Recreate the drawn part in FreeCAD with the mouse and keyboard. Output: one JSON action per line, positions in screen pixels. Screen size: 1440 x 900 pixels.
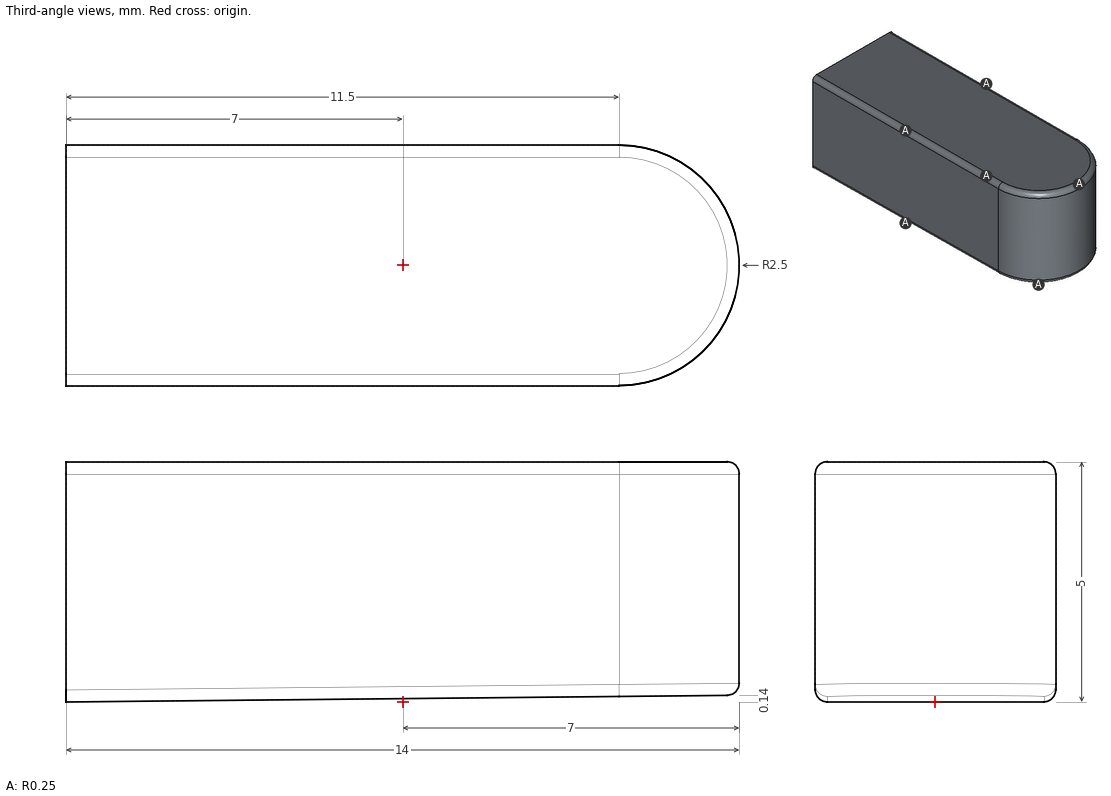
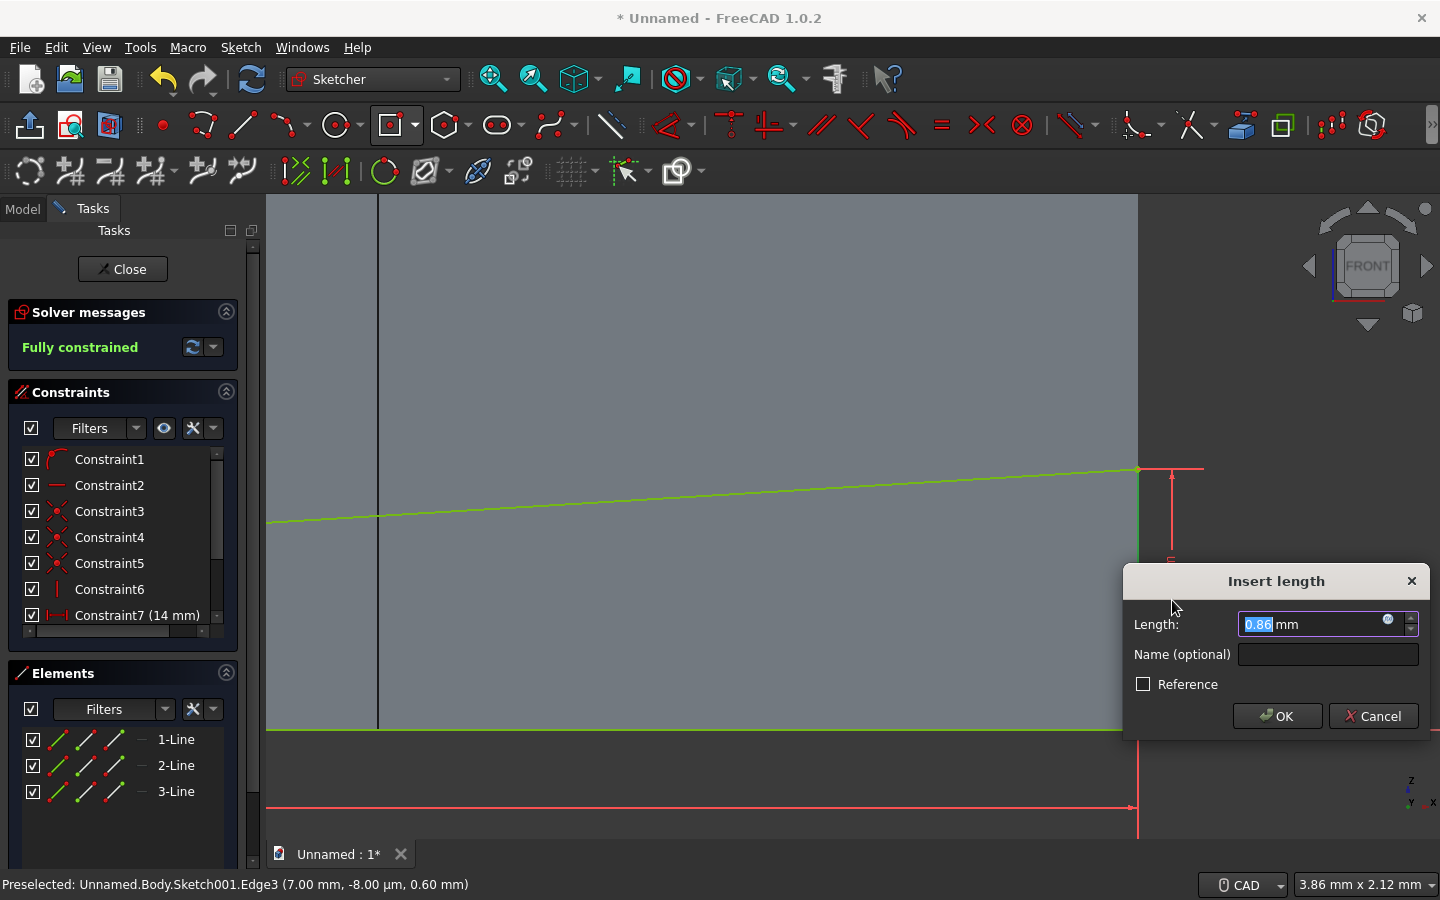
{"action": "type", "text": "0.14"}
{"action": "key", "text": "Return"}
{"action": "key", "text": "Escape"}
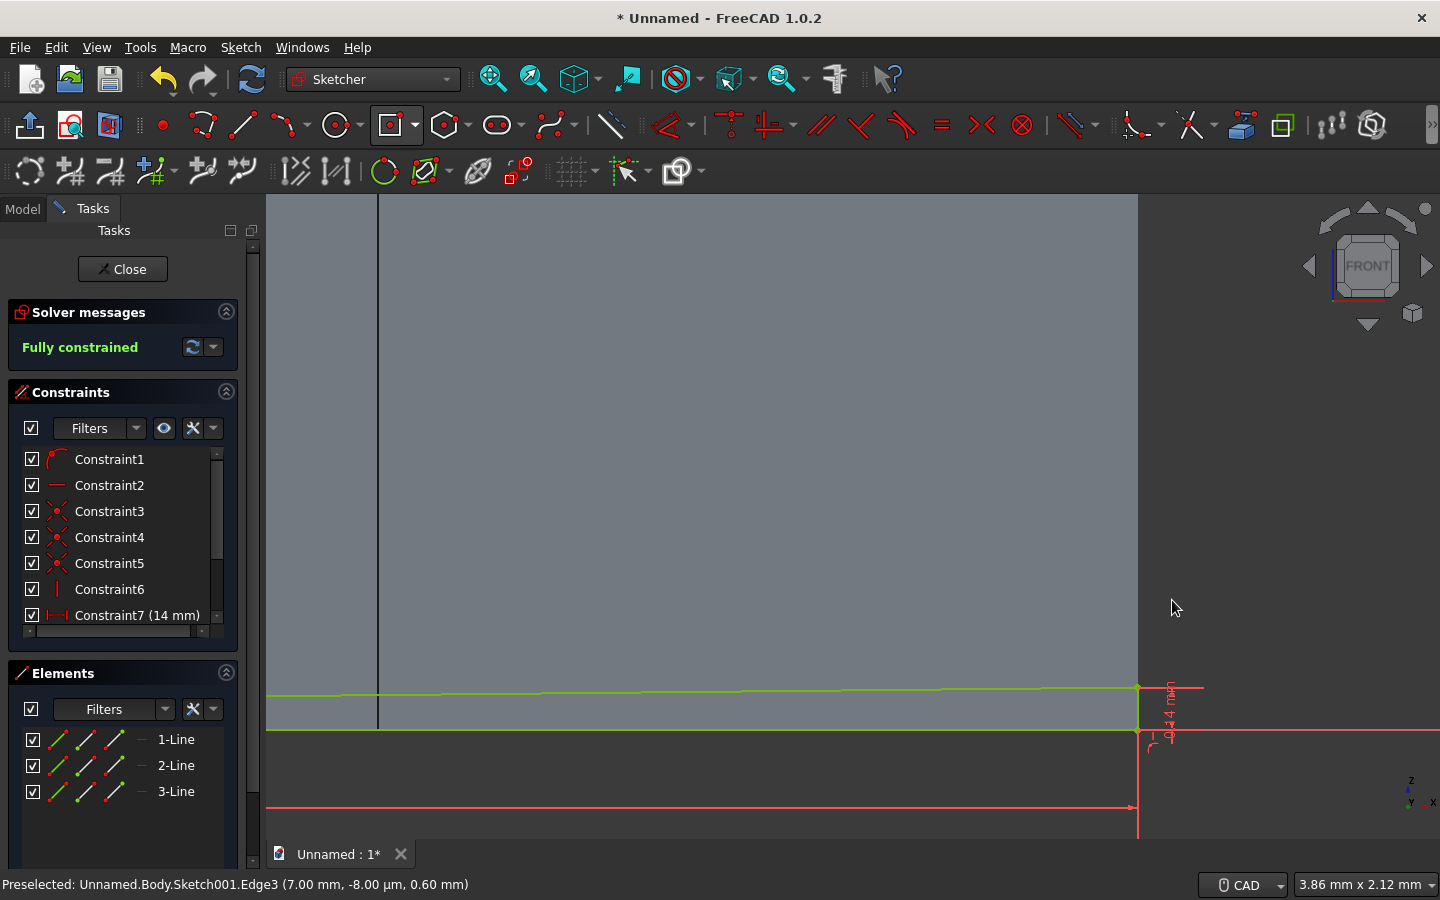
{"action": "left_click", "coordinate": [123, 269]}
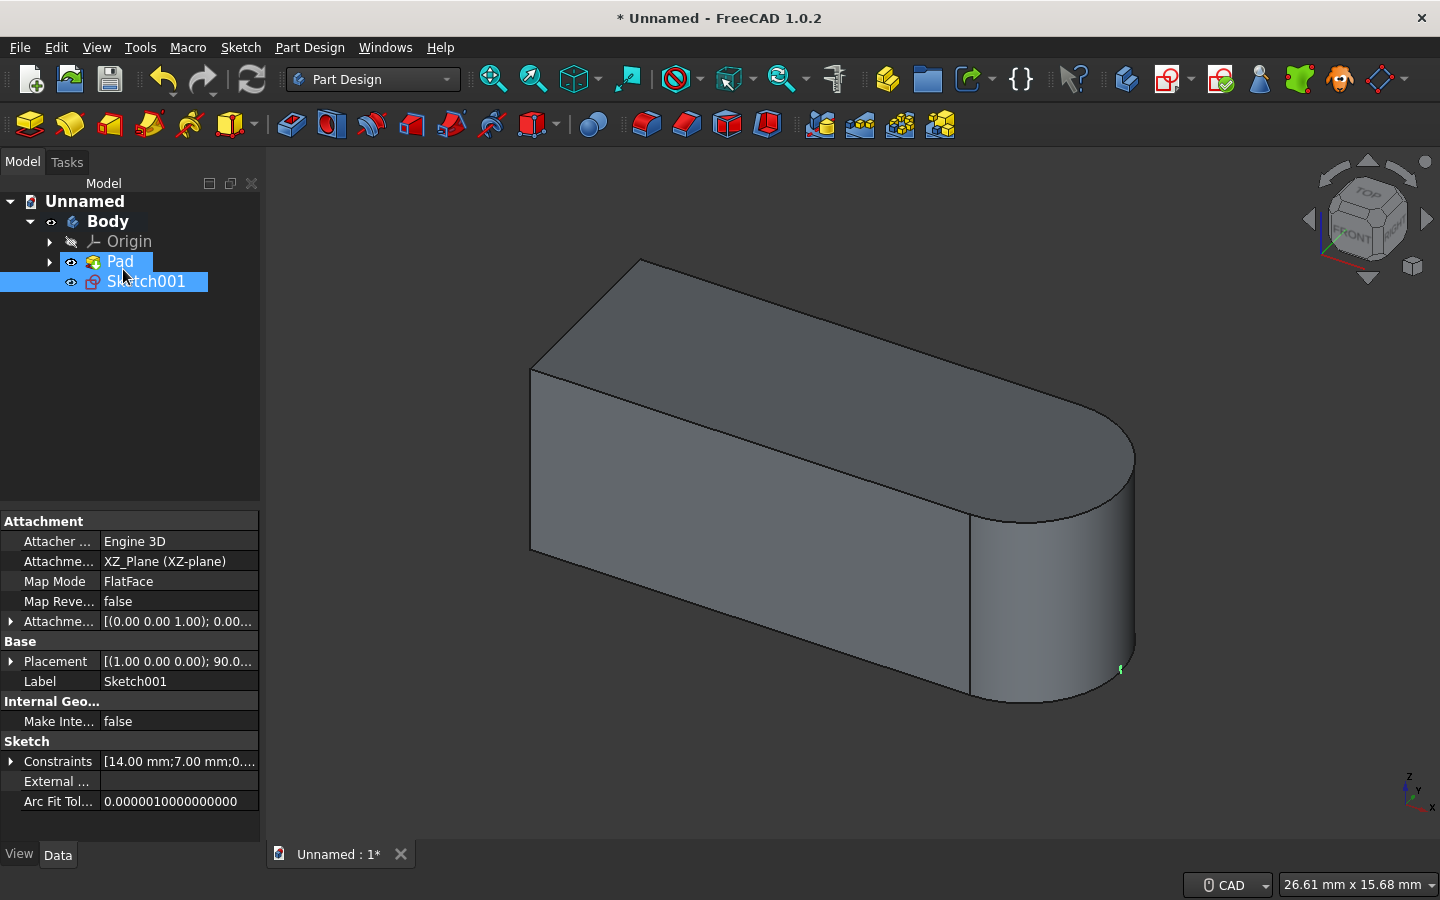
{"action": "left_click", "coordinate": [292, 124]}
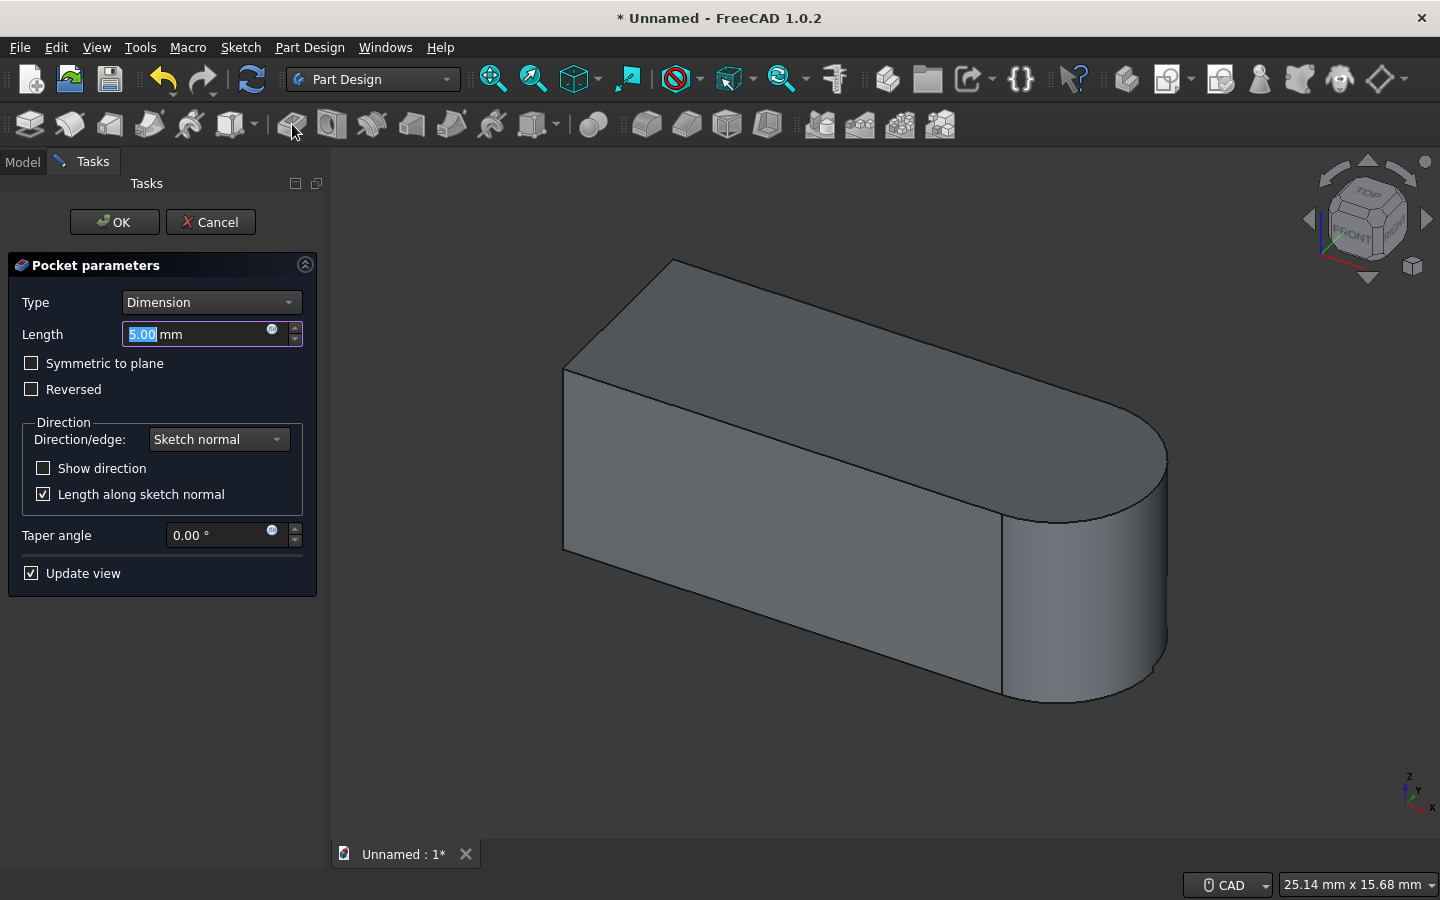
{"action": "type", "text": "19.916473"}
{"action": "key", "text": "Tab"}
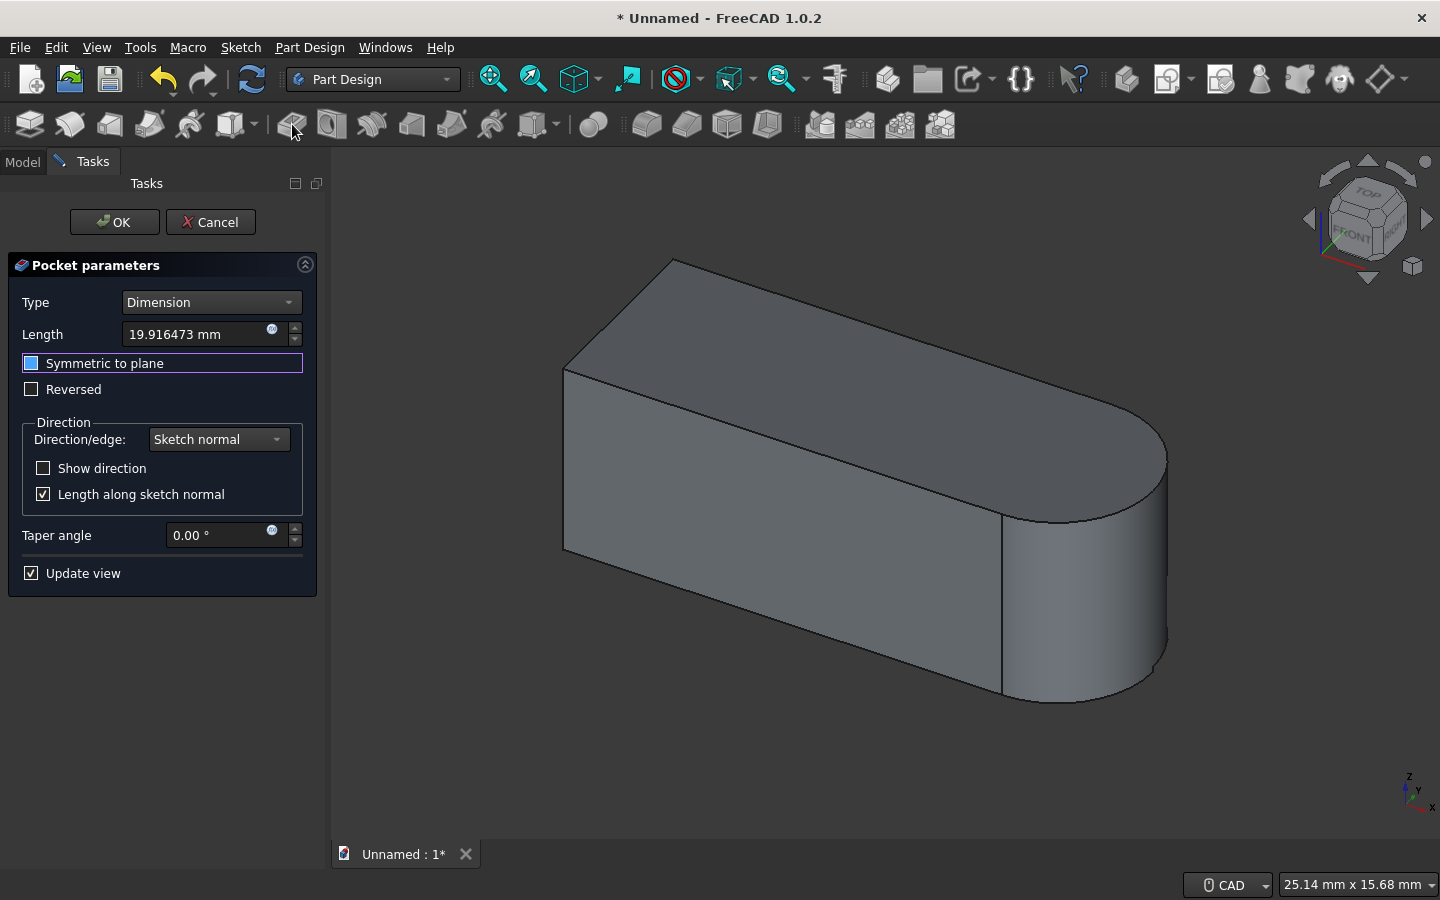
{"action": "left_click", "coordinate": [30, 363]}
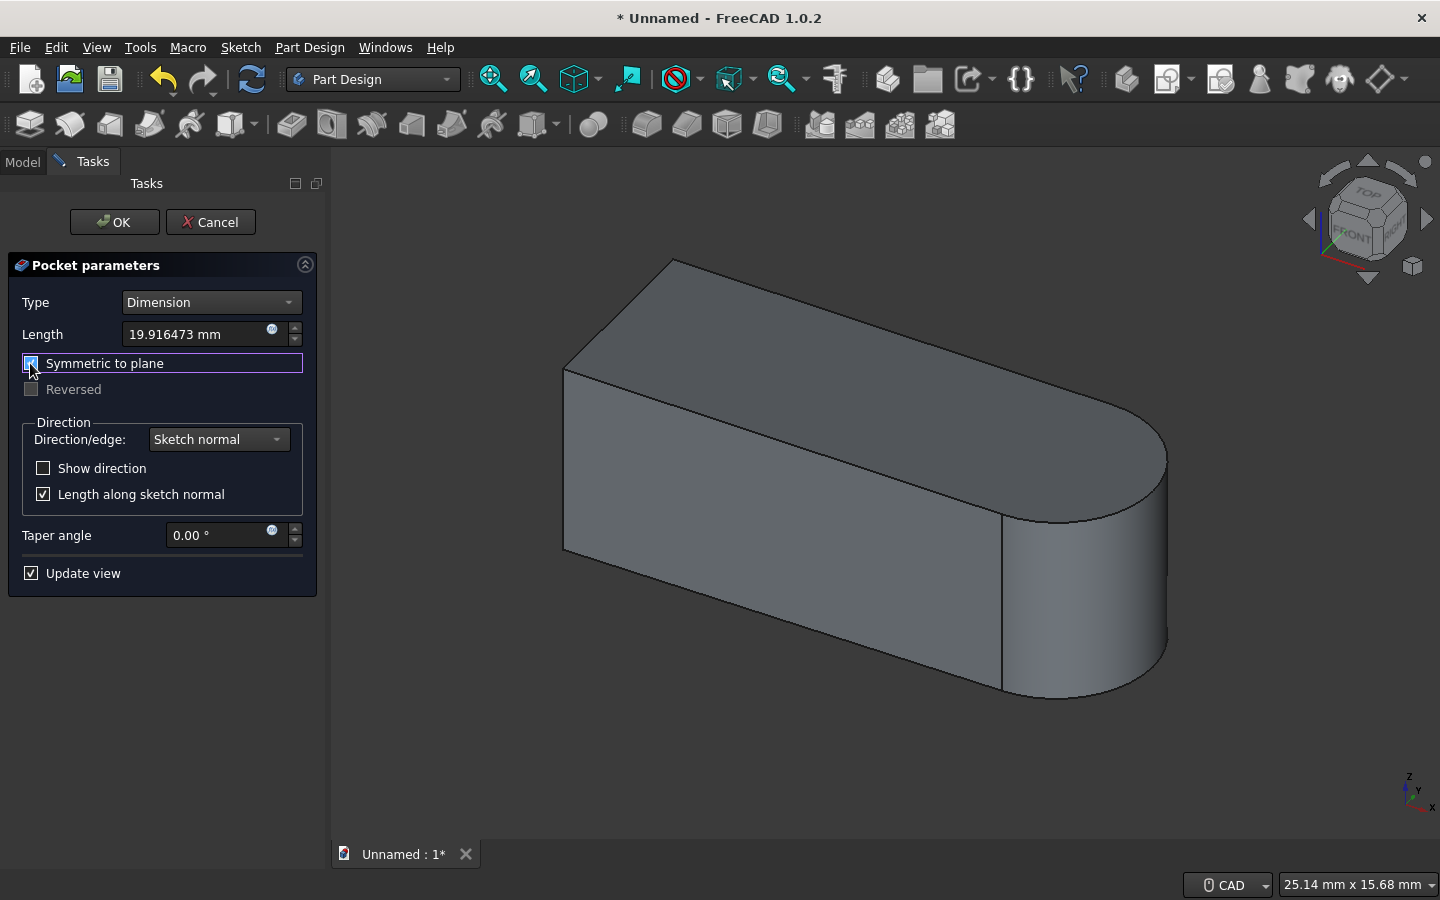
{"action": "left_click", "coordinate": [115, 222]}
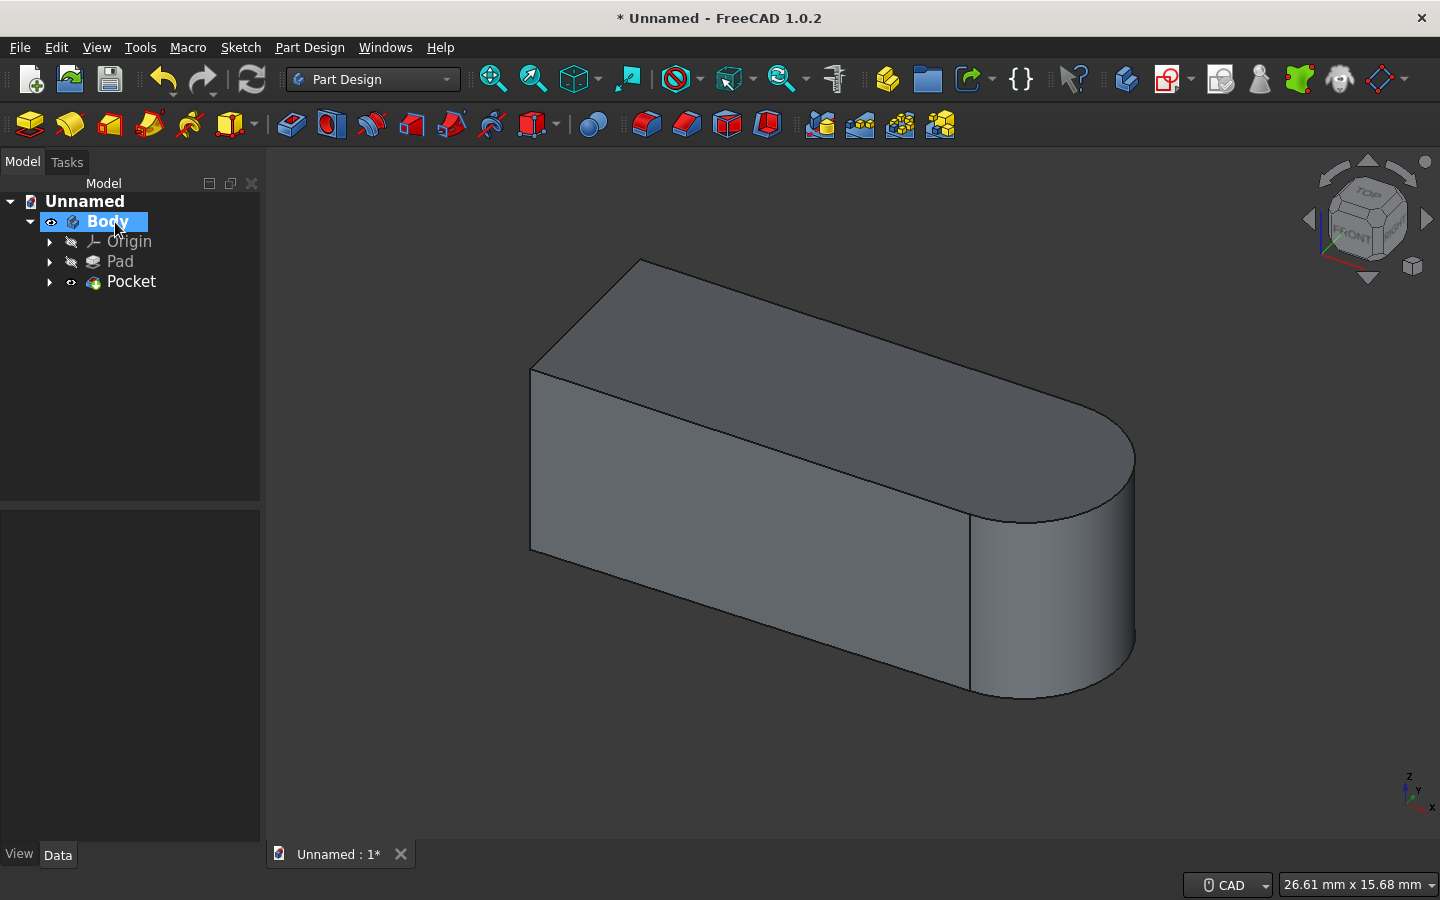
{"action": "left_click", "coordinate": [1120, 490]}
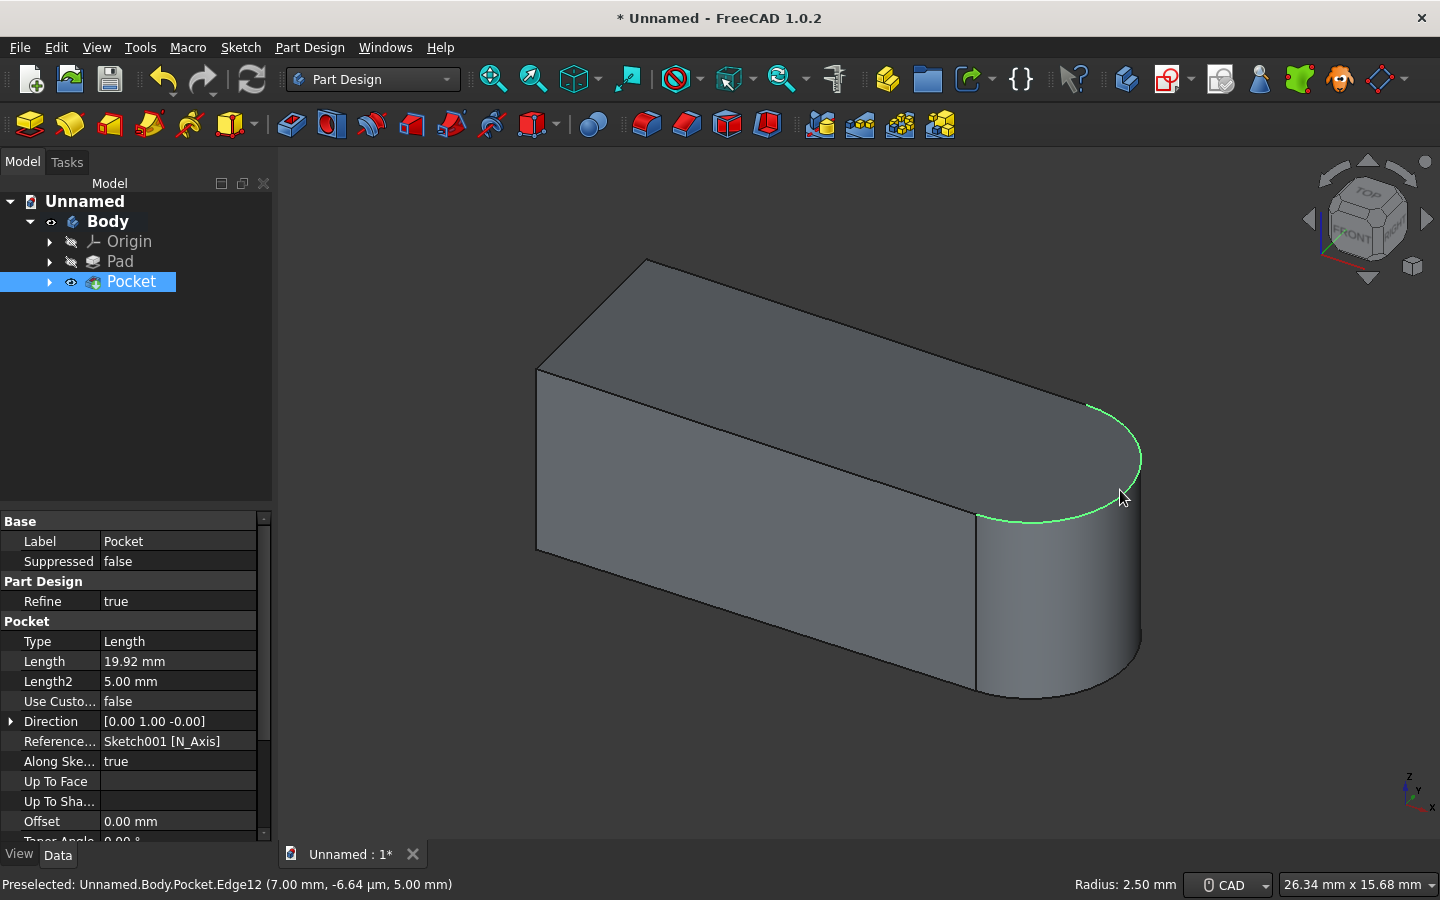
{"action": "left_click", "coordinate": [756, 441], "text": "ctrl"}